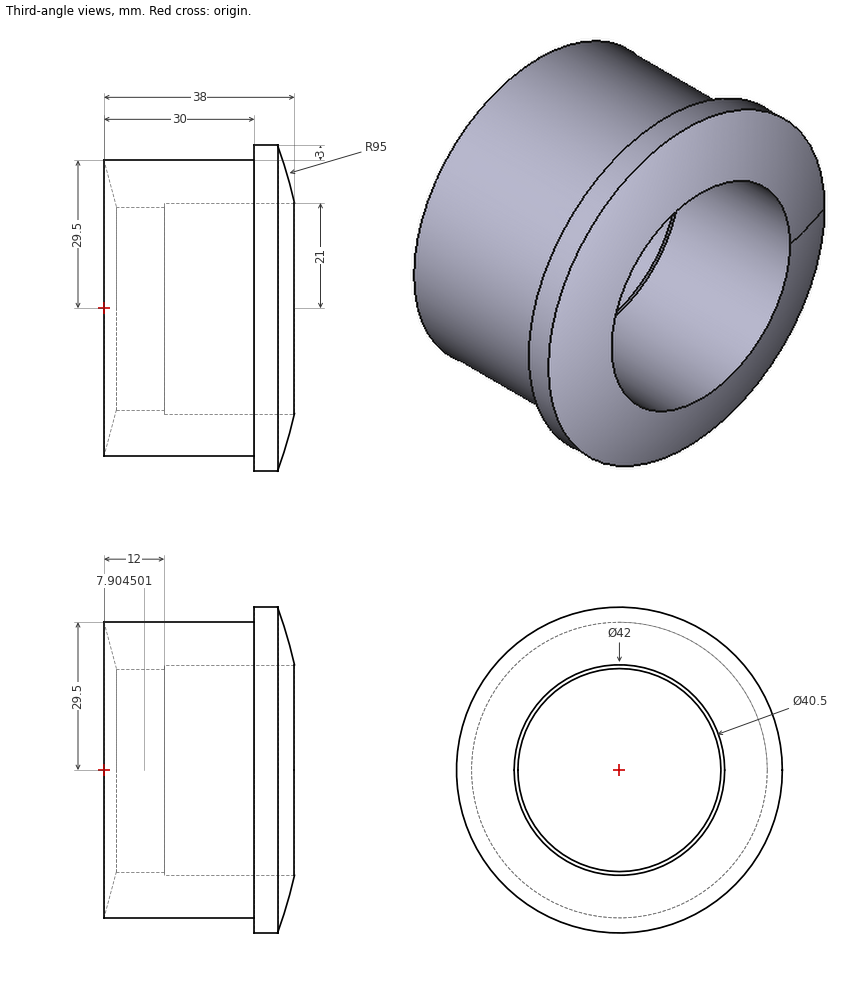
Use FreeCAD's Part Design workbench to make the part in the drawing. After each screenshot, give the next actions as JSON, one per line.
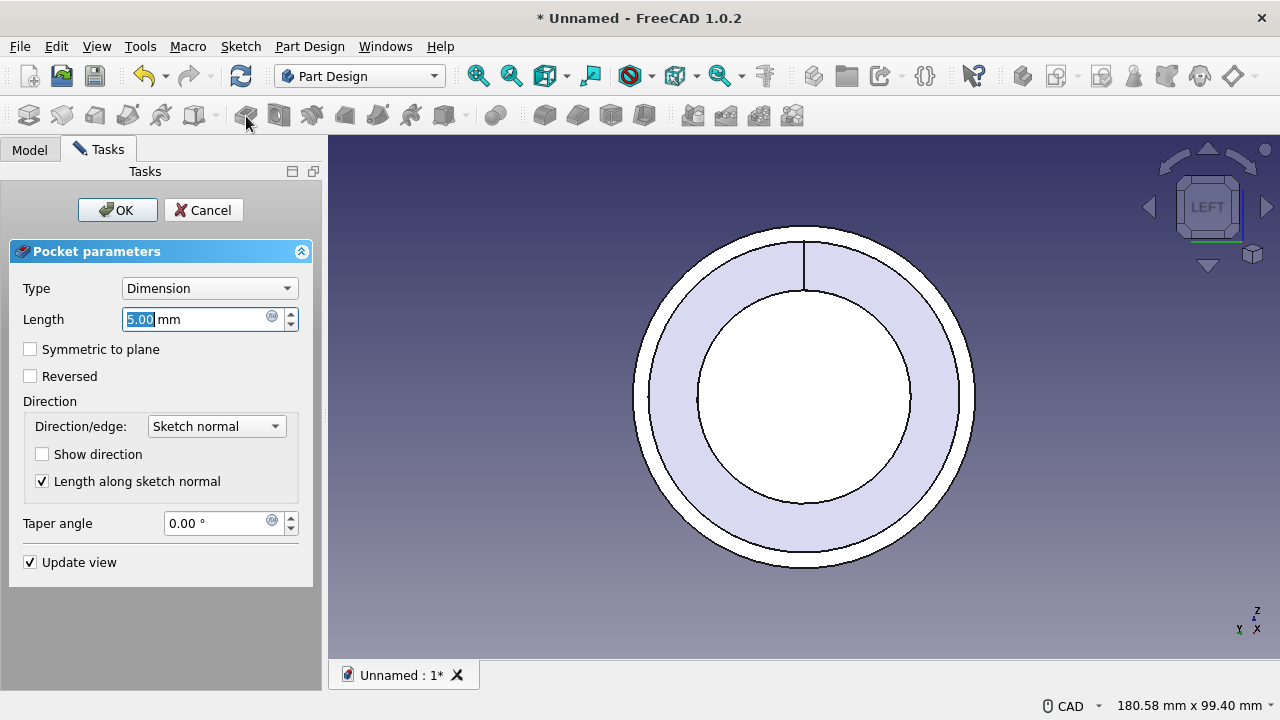
{"action": "left_click", "coordinate": [210, 288]}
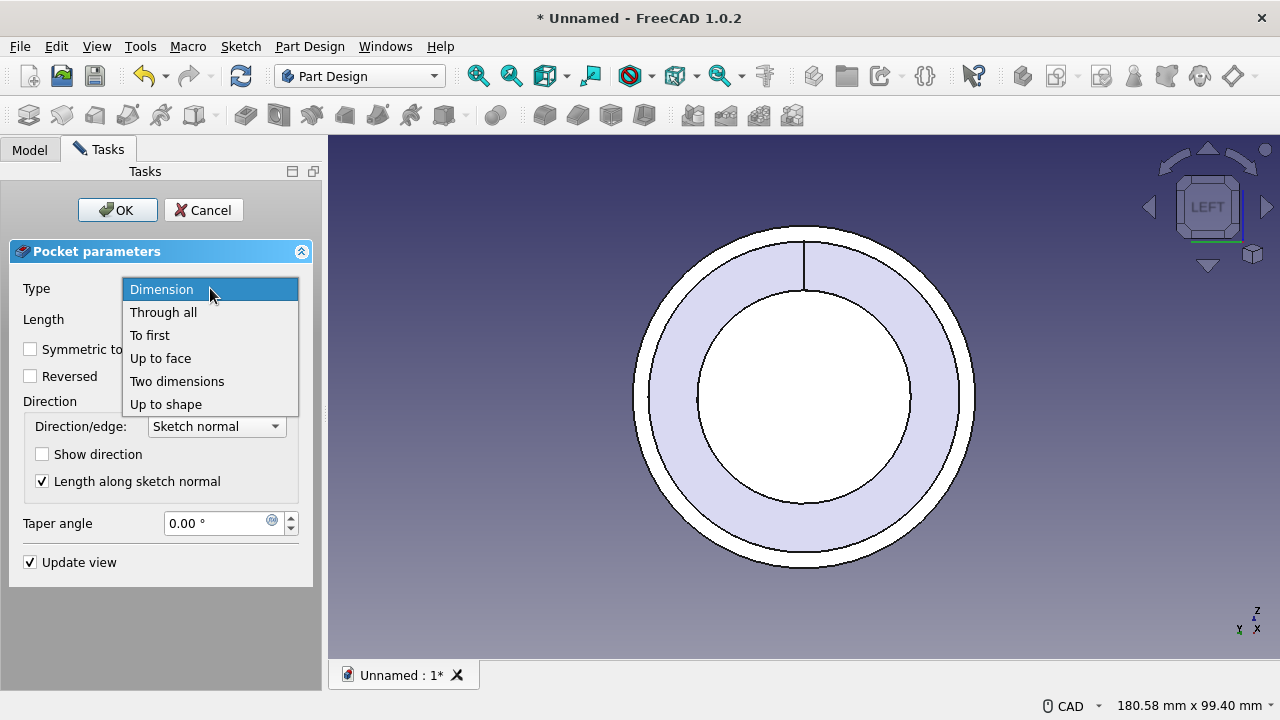
{"action": "left_click", "coordinate": [208, 312]}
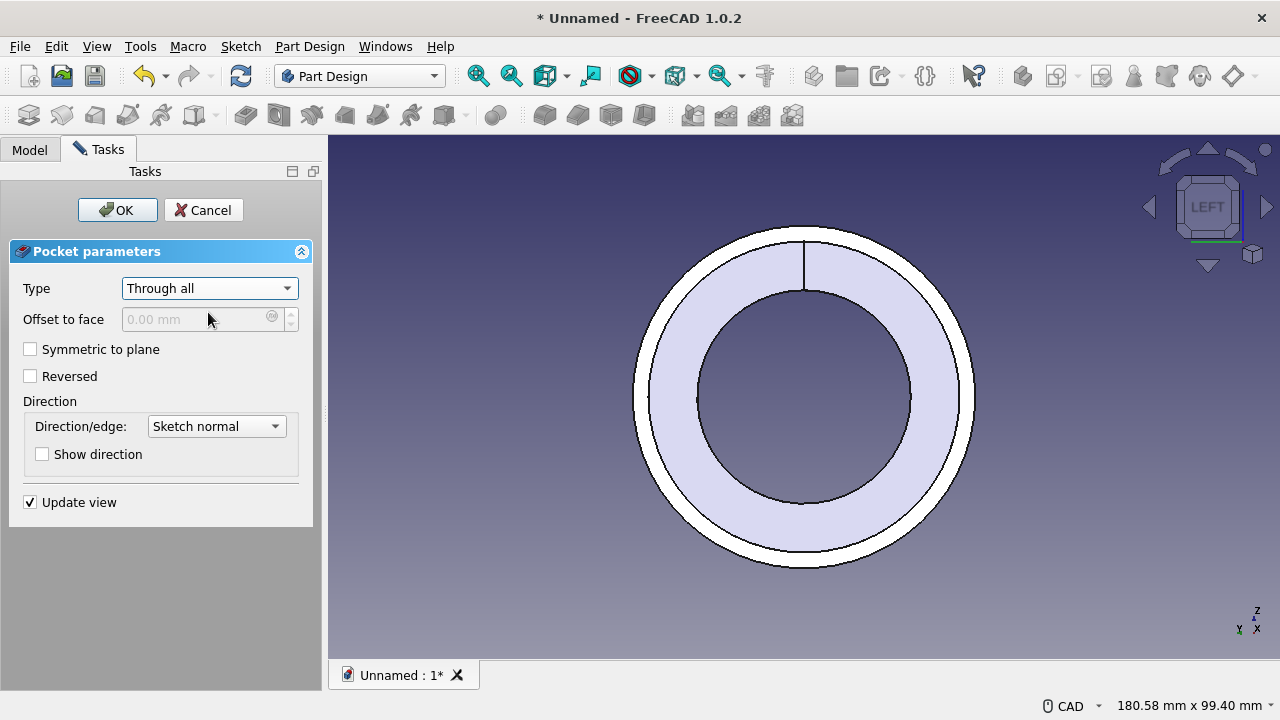
{"action": "left_click", "coordinate": [118, 210]}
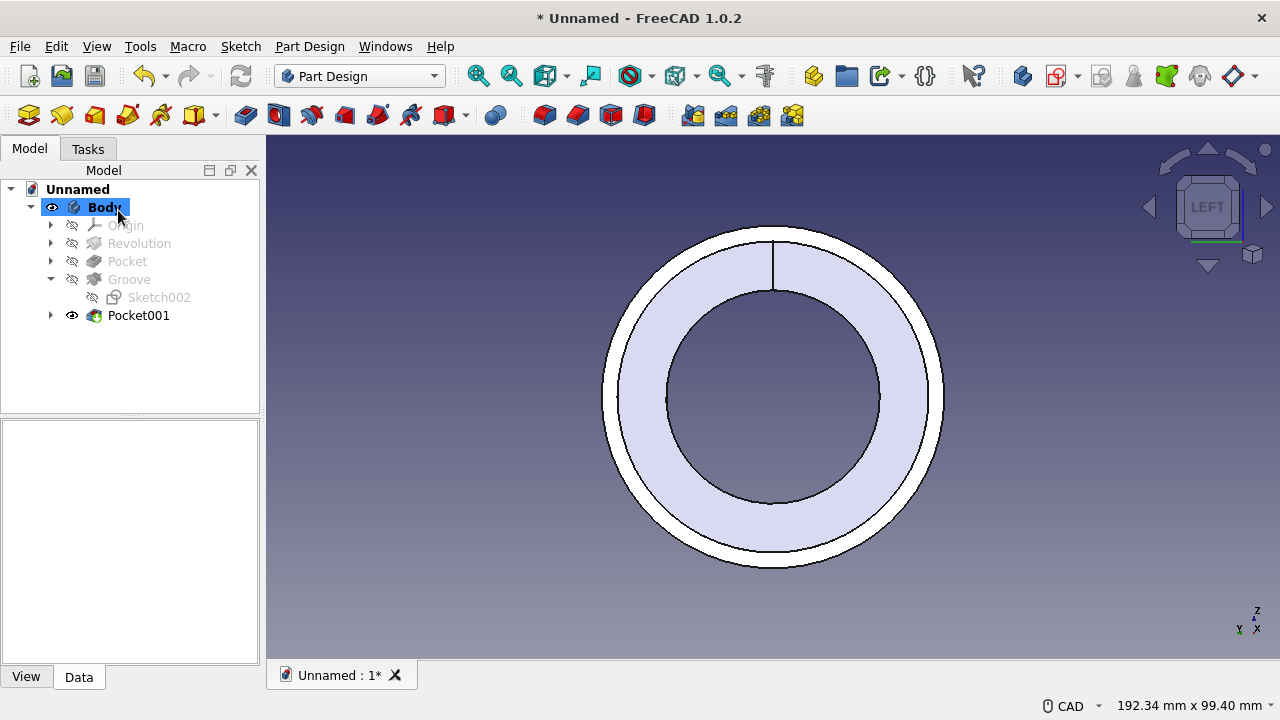
{"action": "key", "text": "0"}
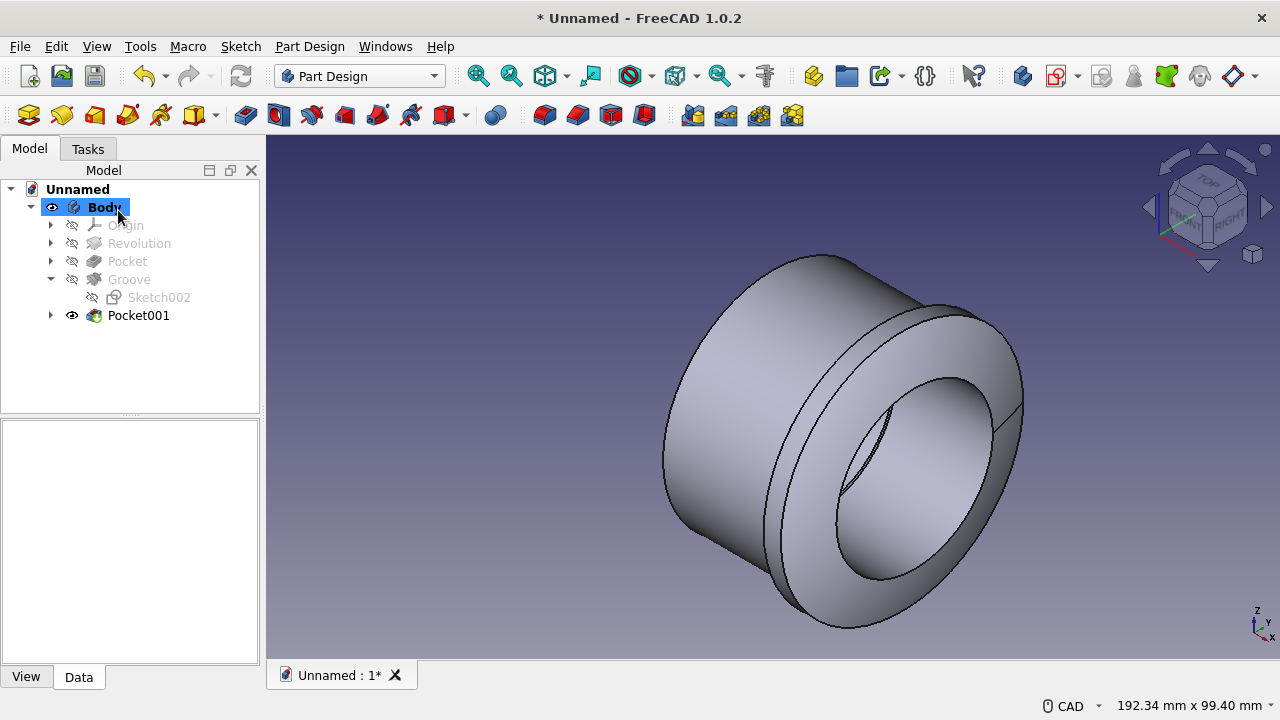
{"action": "left_click", "coordinate": [479, 76]}